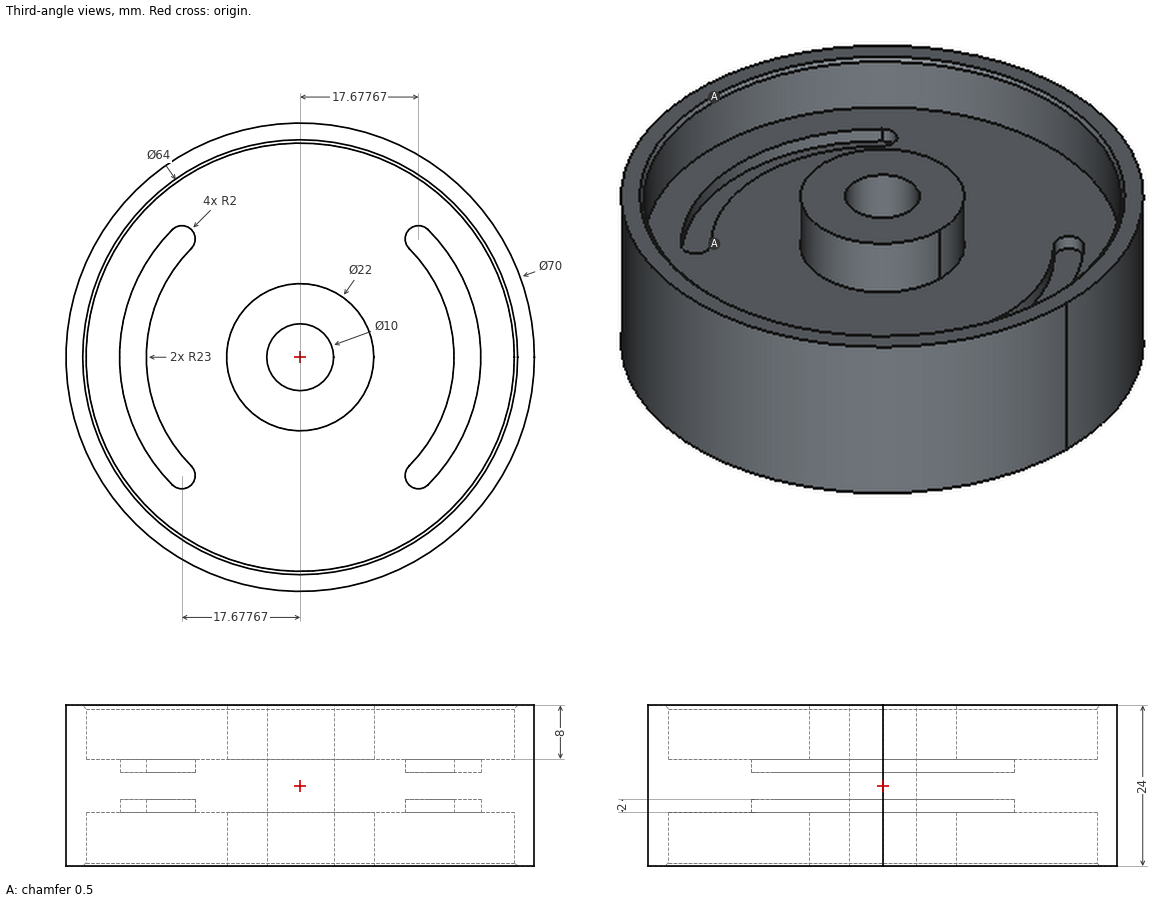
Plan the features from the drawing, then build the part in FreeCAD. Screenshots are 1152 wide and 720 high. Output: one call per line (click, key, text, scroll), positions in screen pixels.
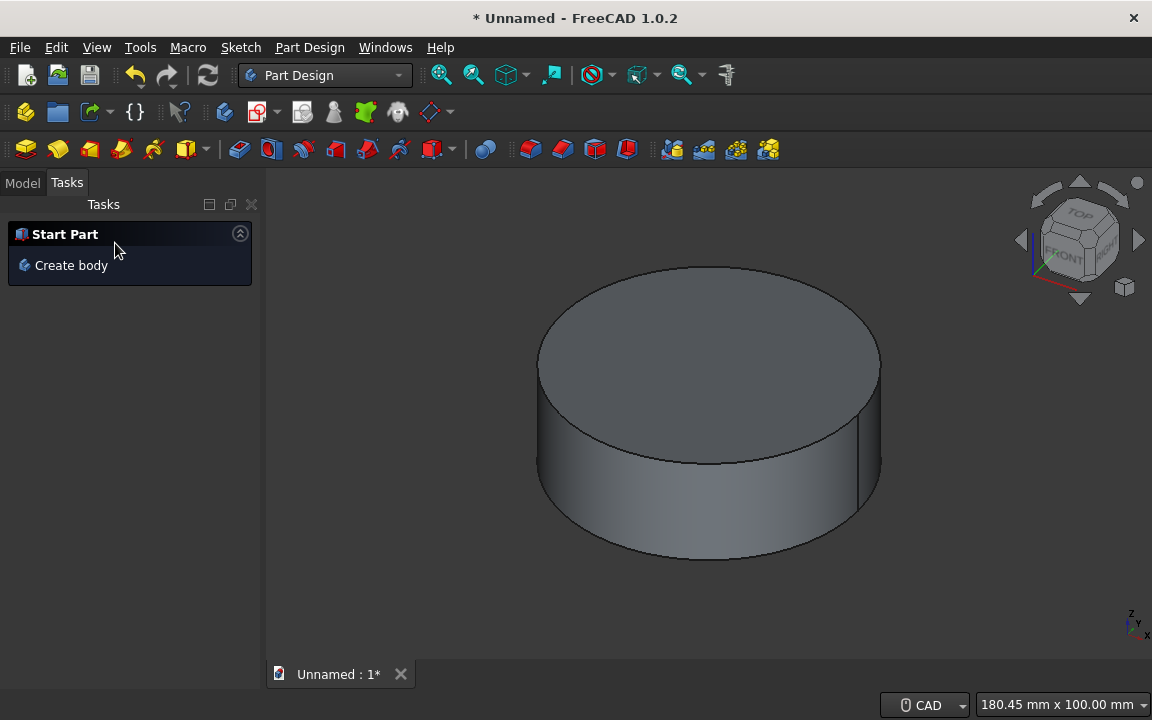
click(709, 364)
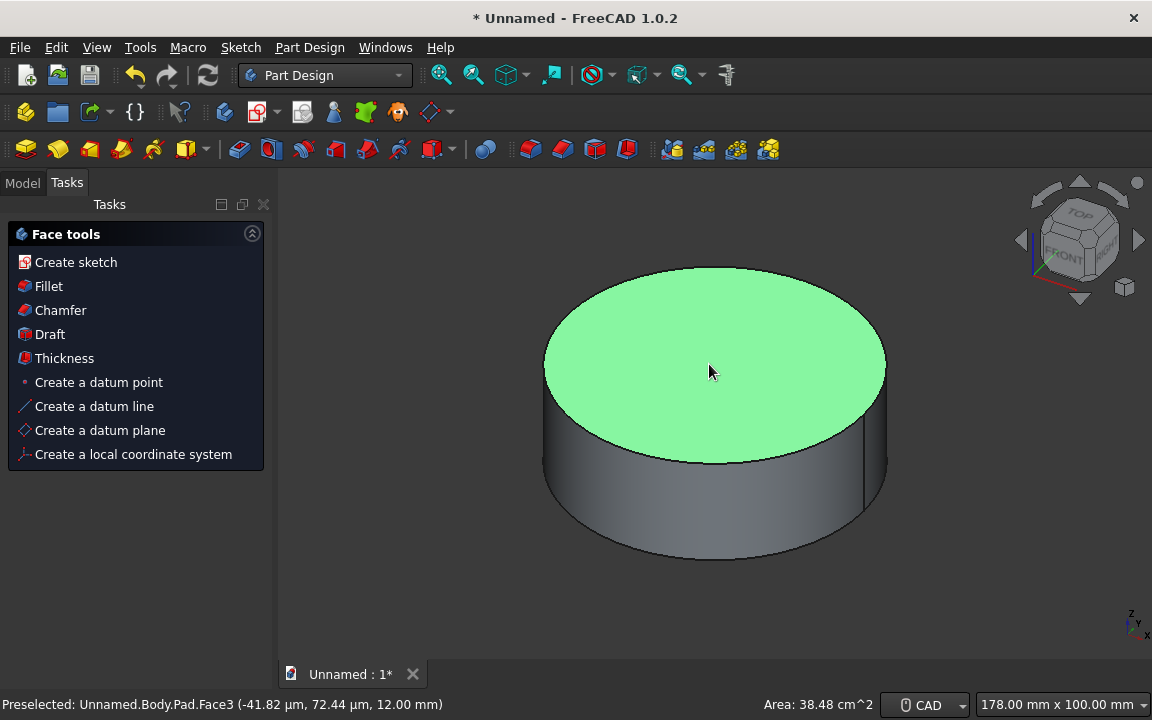
click(258, 112)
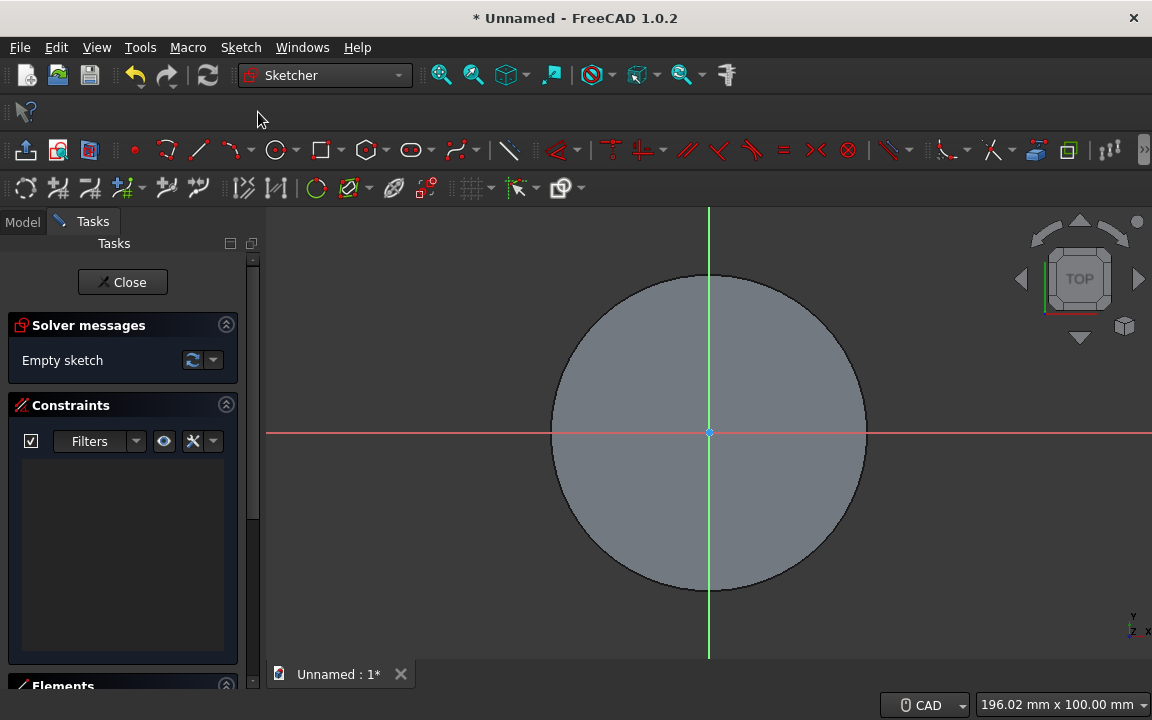
scroll(723, 433, up, 9)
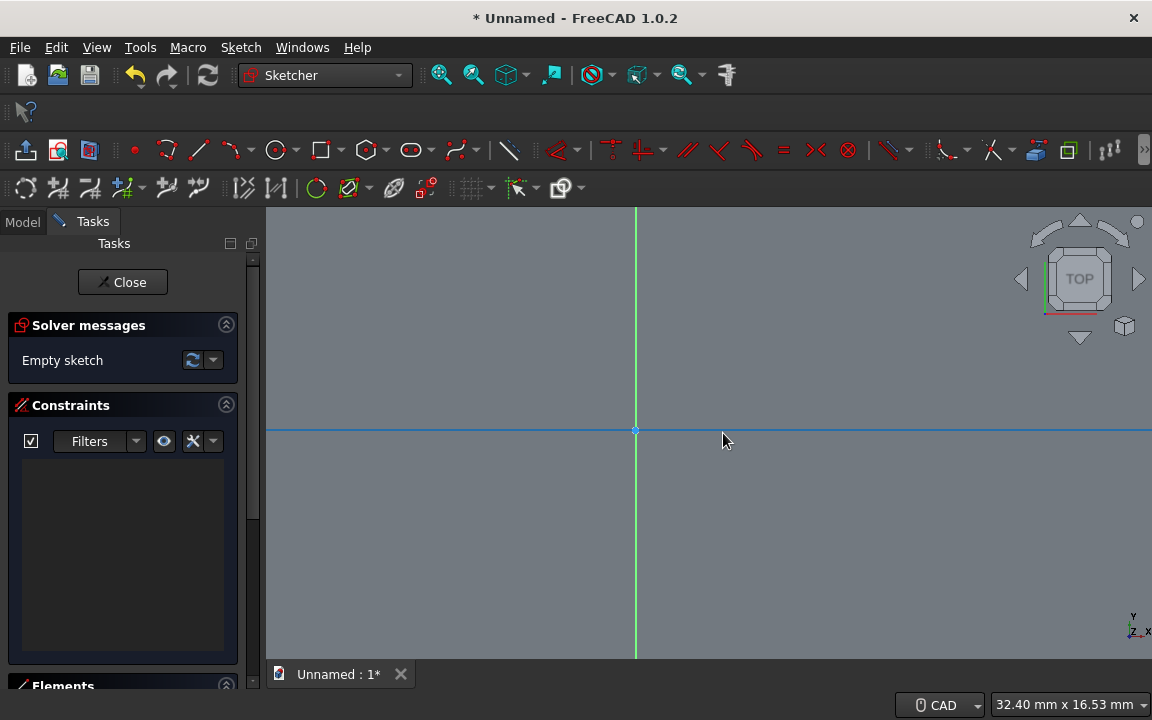
key(g)
key(c)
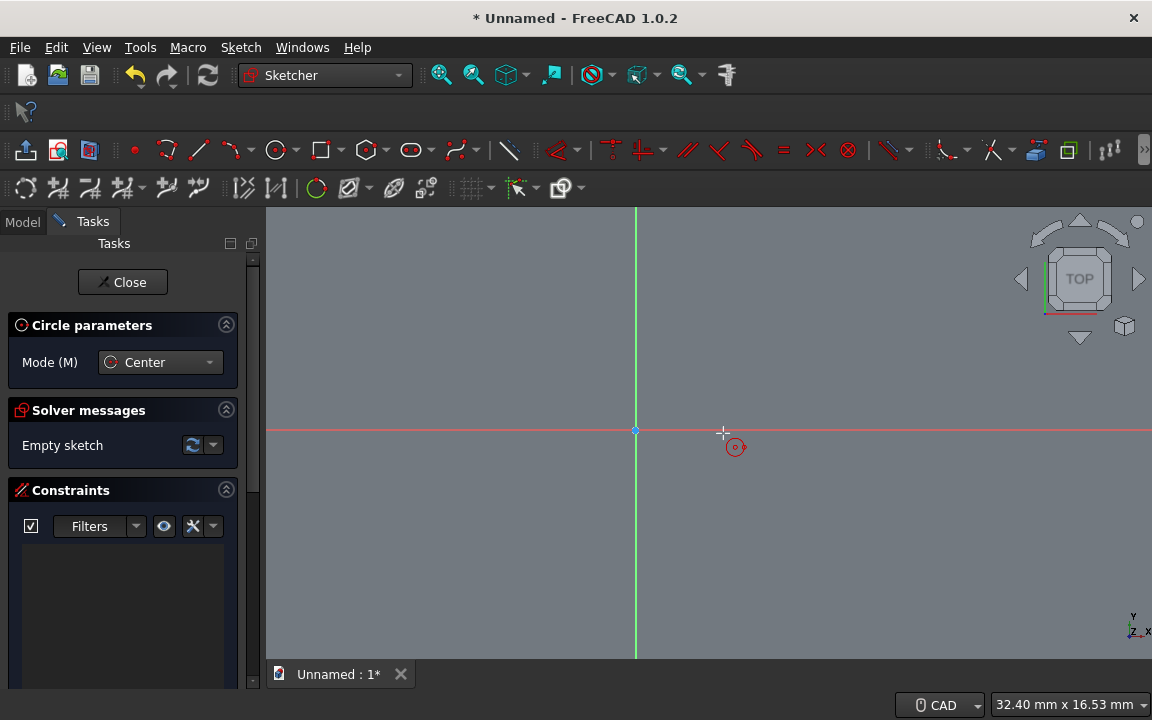
click(636, 430)
move(732, 334)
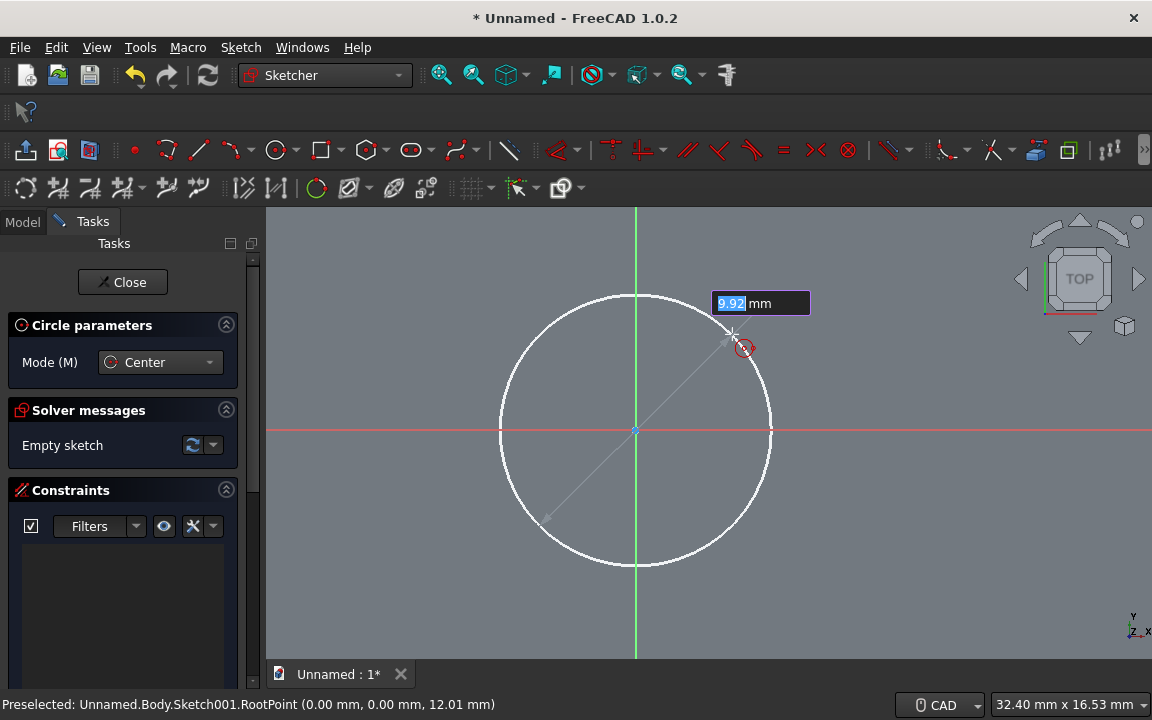
text(10)
key(Return)
key(Escape)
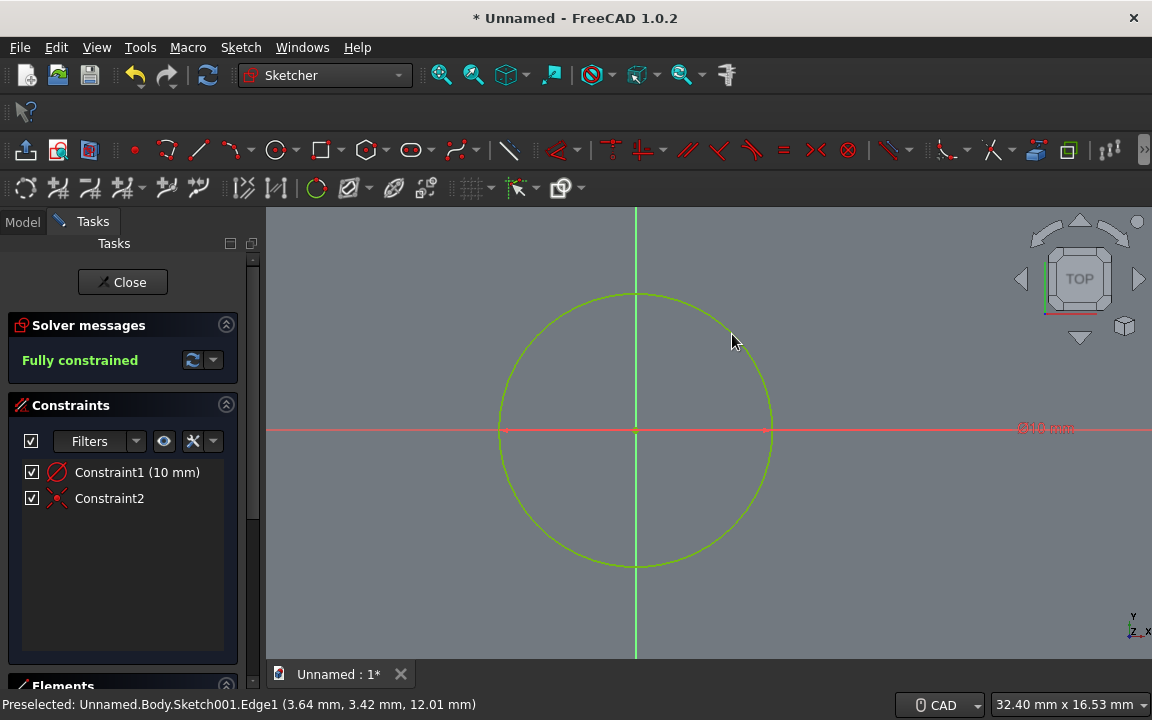
click(123, 282)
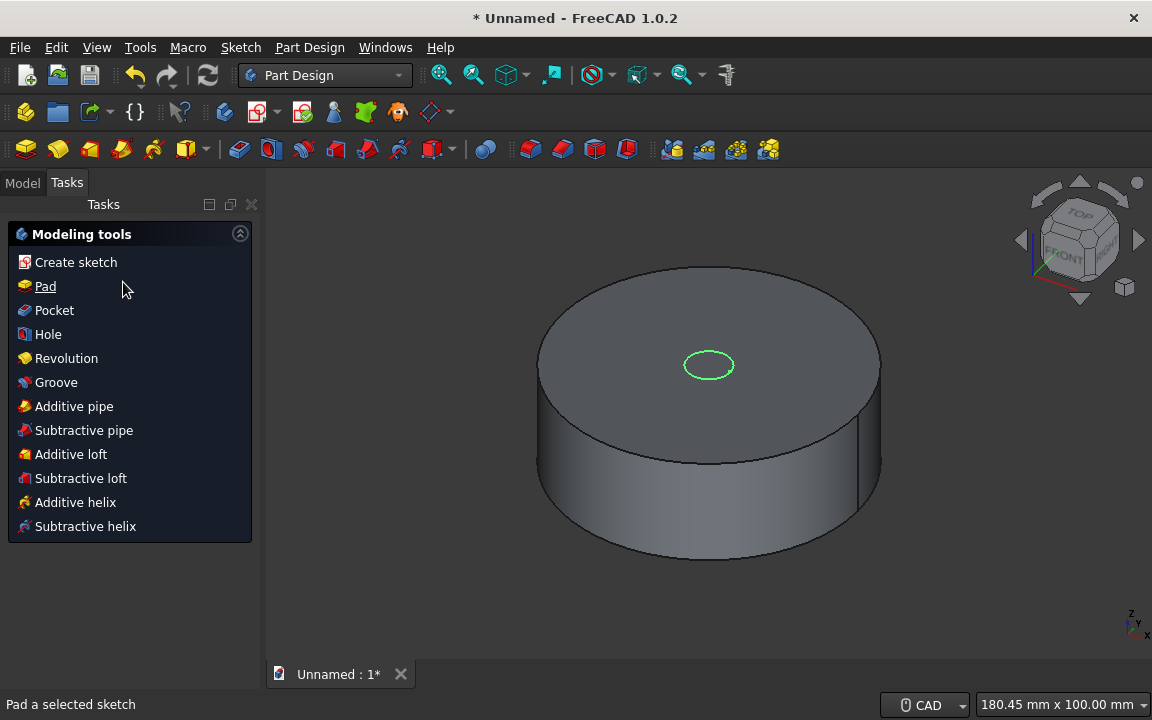
click(240, 150)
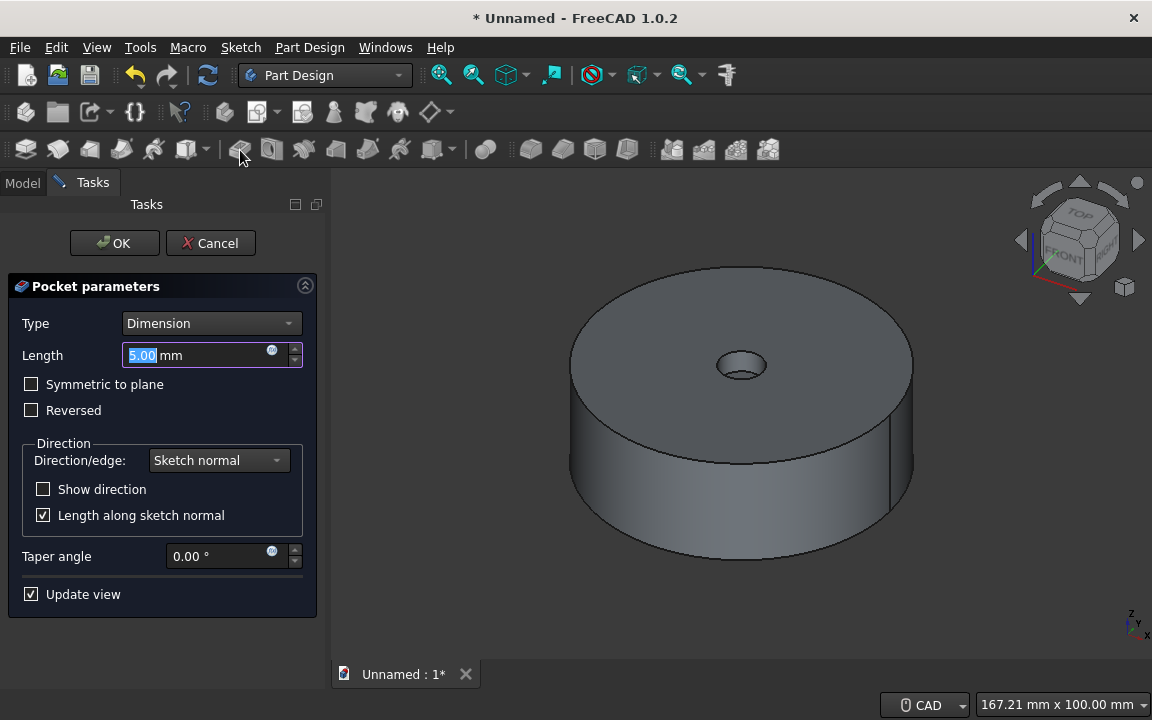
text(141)
key(Tab)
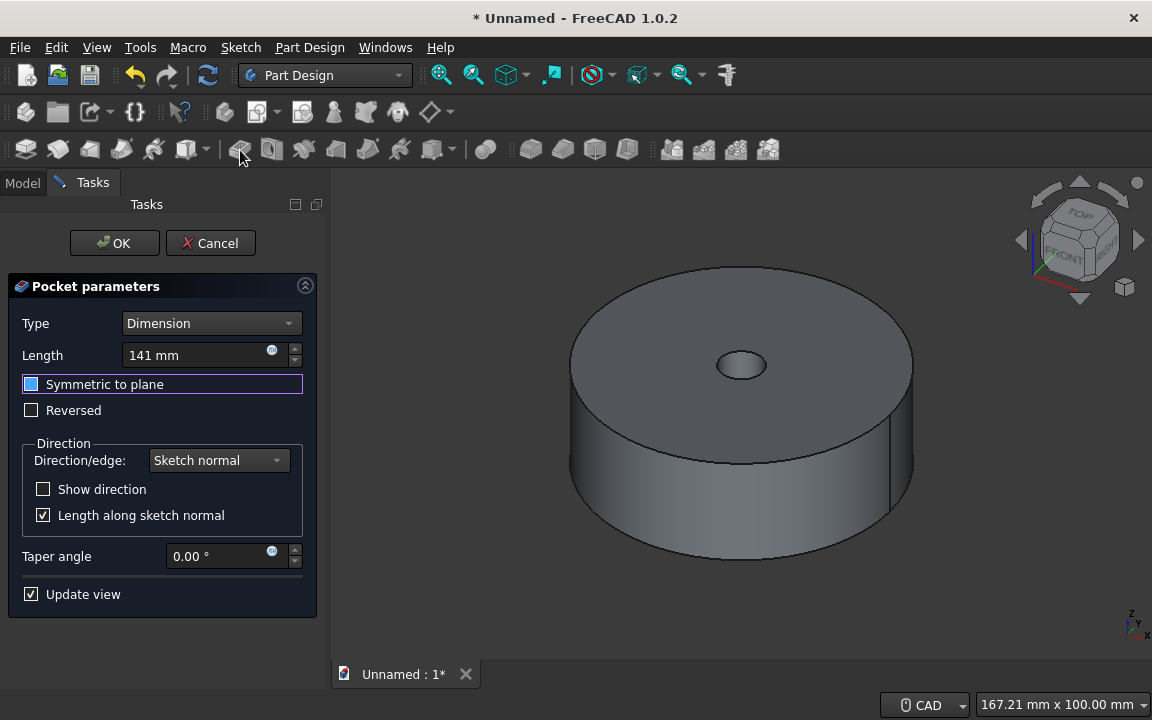
click(30, 384)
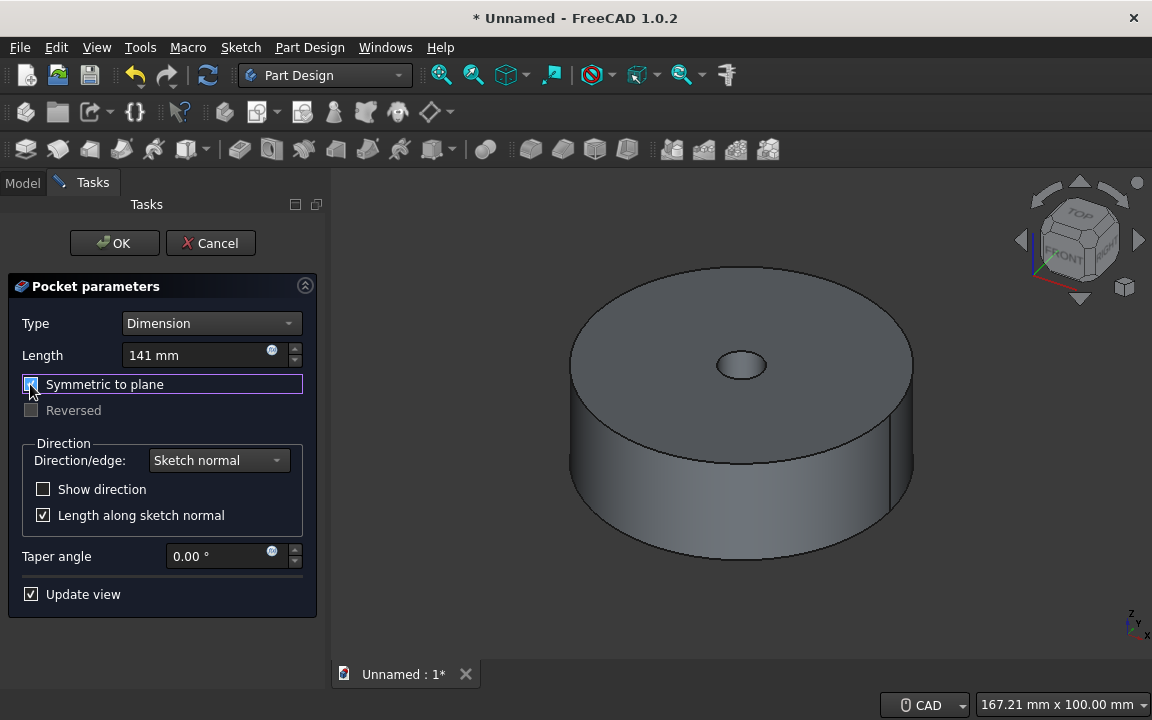
click(115, 243)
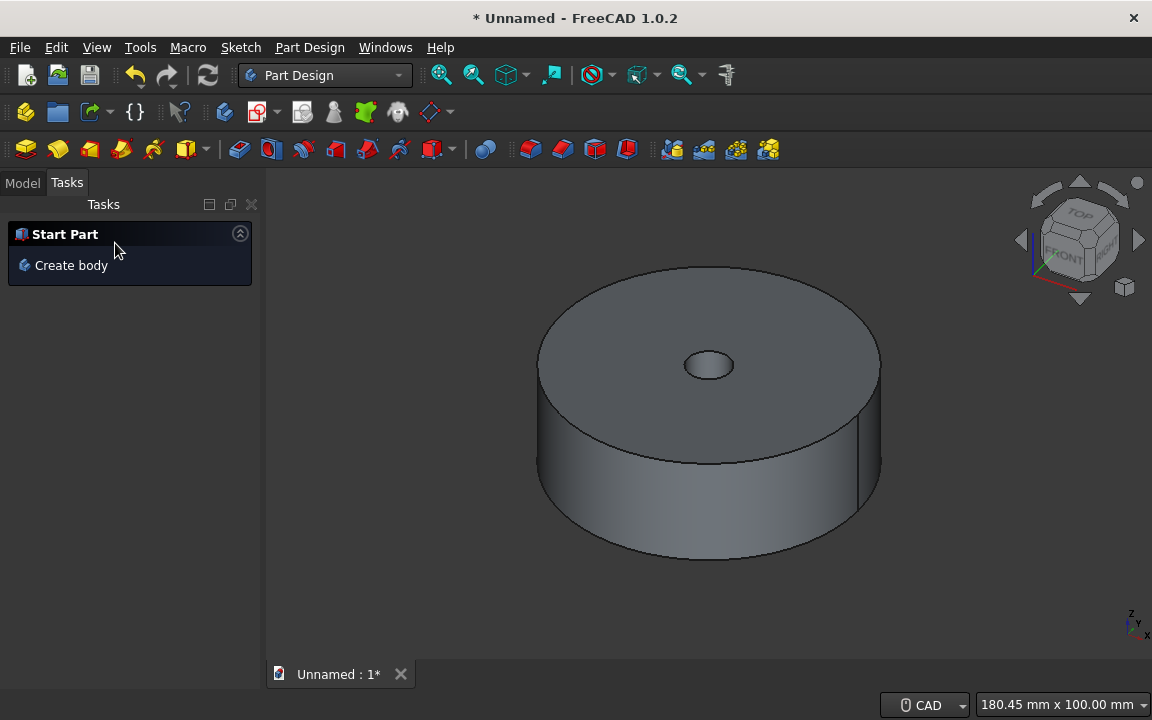
click(794, 392)